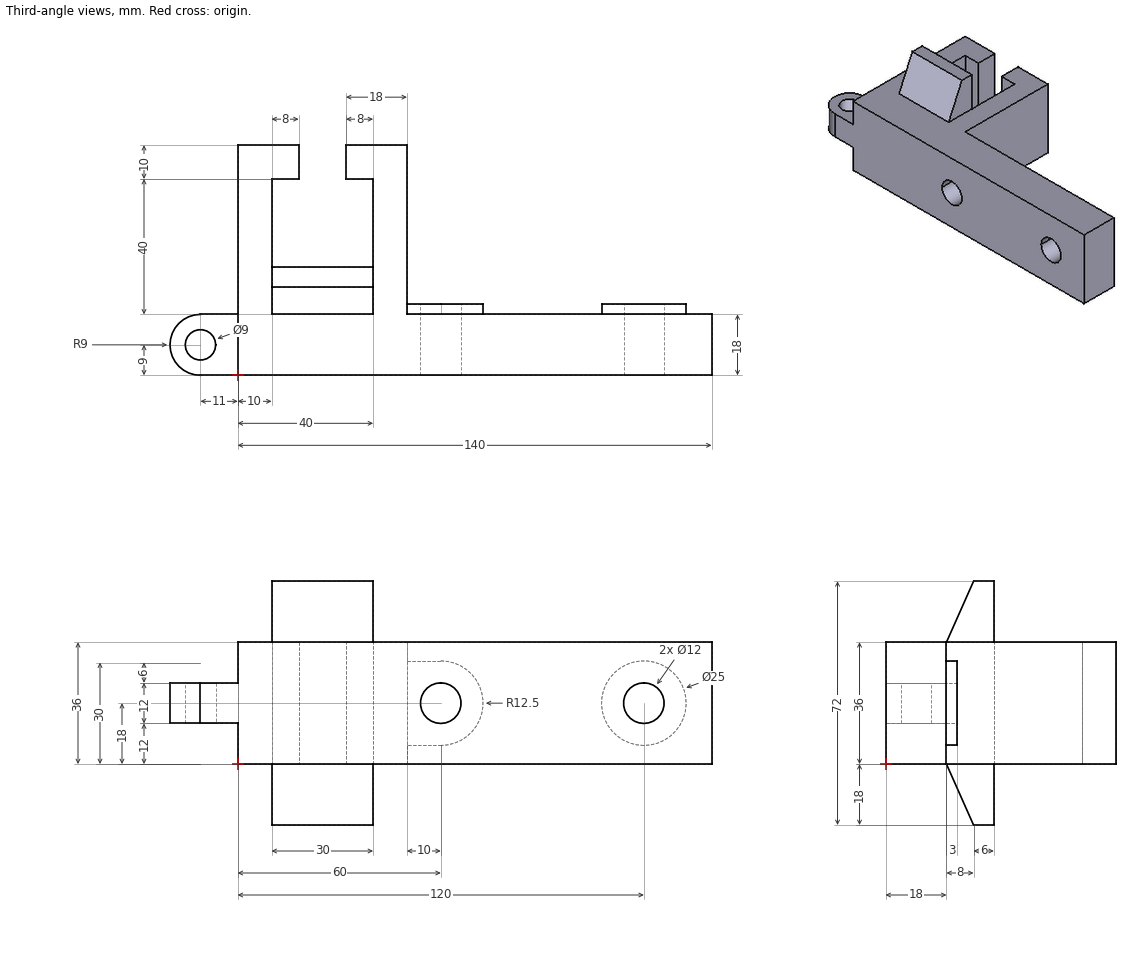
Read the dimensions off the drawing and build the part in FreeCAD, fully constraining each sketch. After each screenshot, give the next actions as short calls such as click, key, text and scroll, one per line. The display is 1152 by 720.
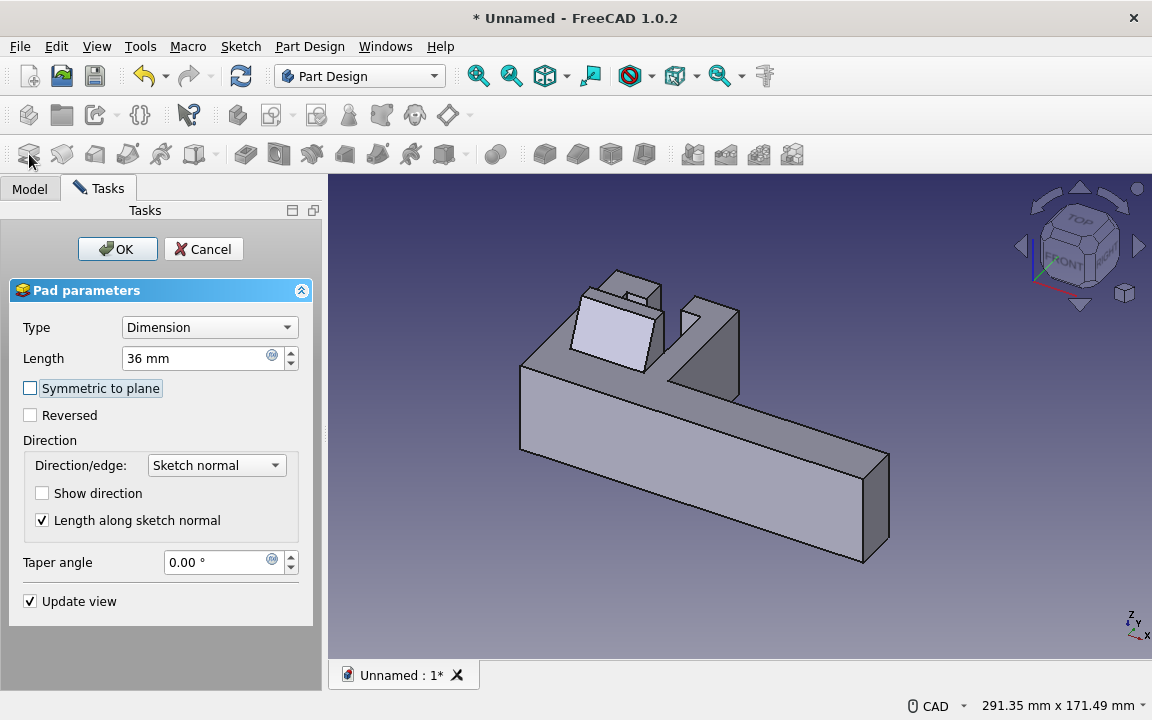
click(118, 249)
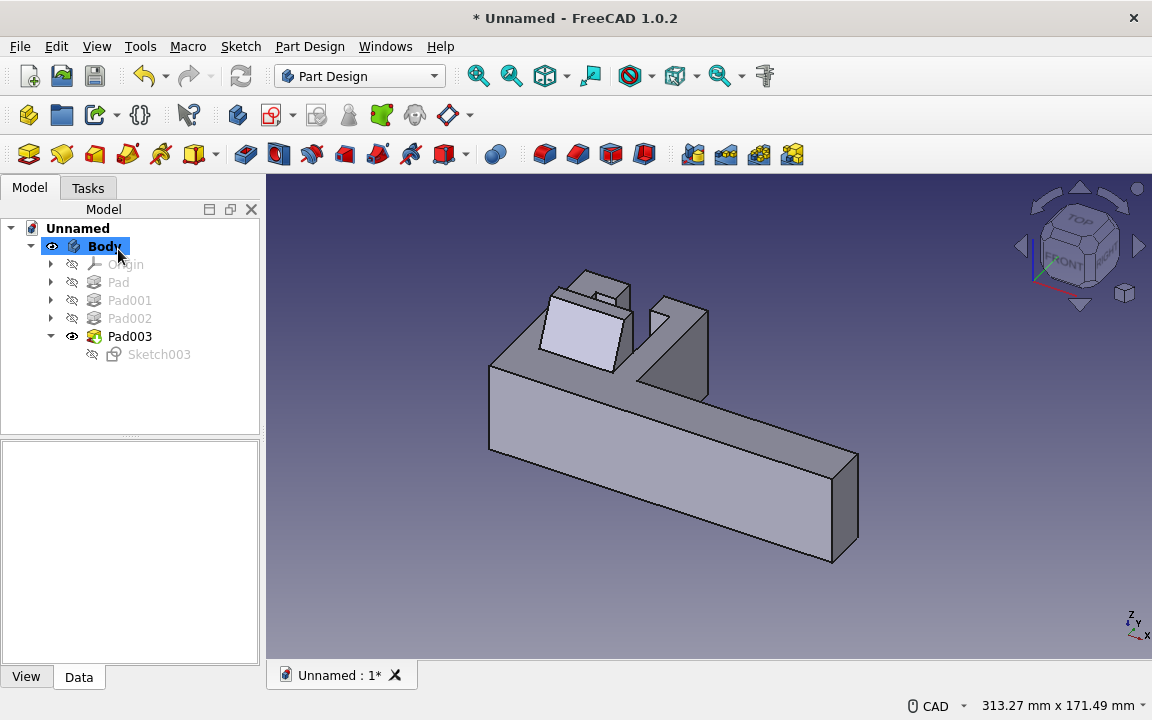
key(5)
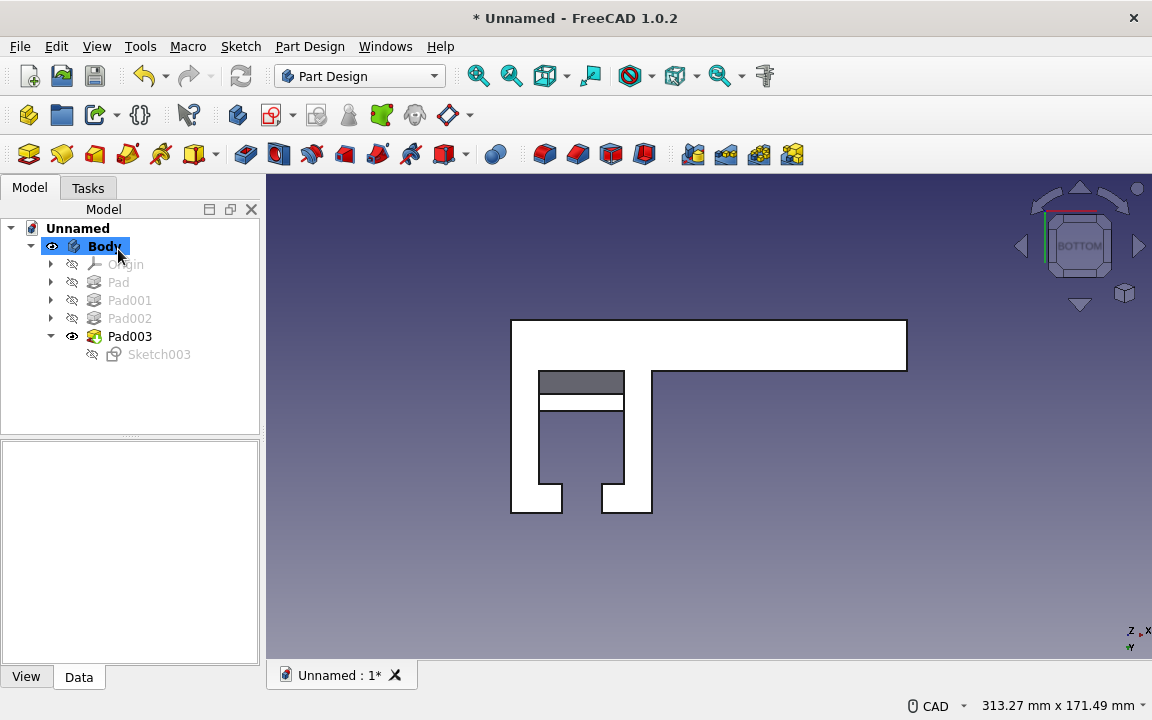
key(v)
key(f)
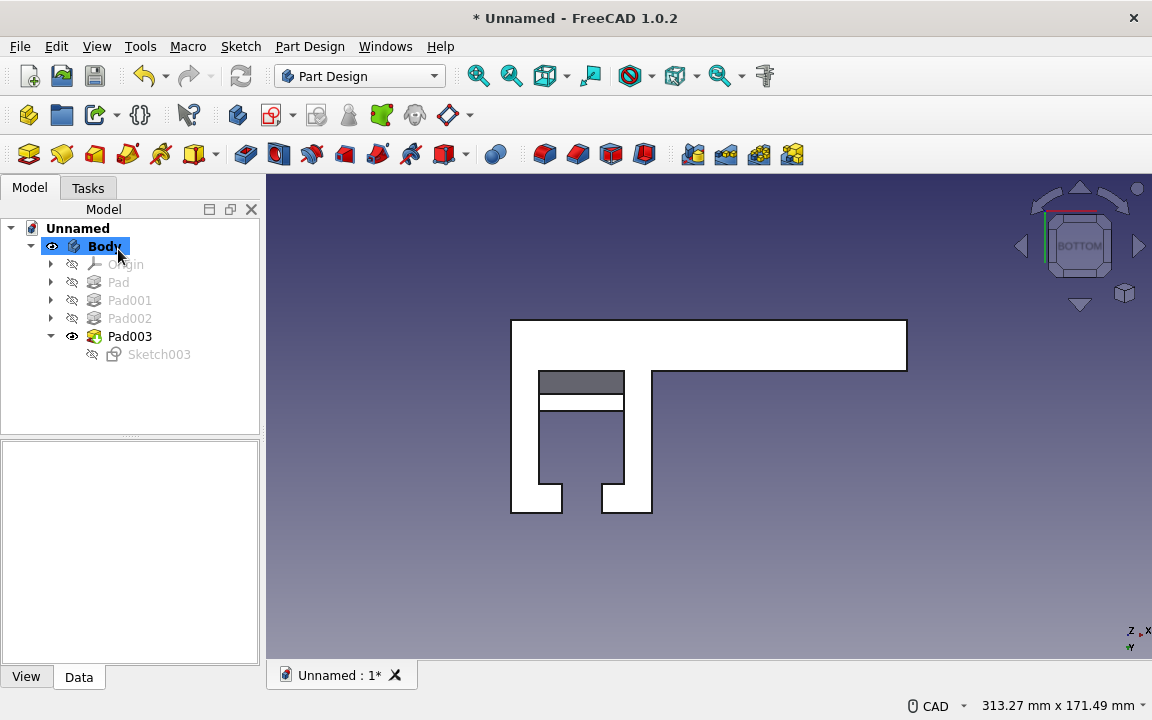
click(879, 333)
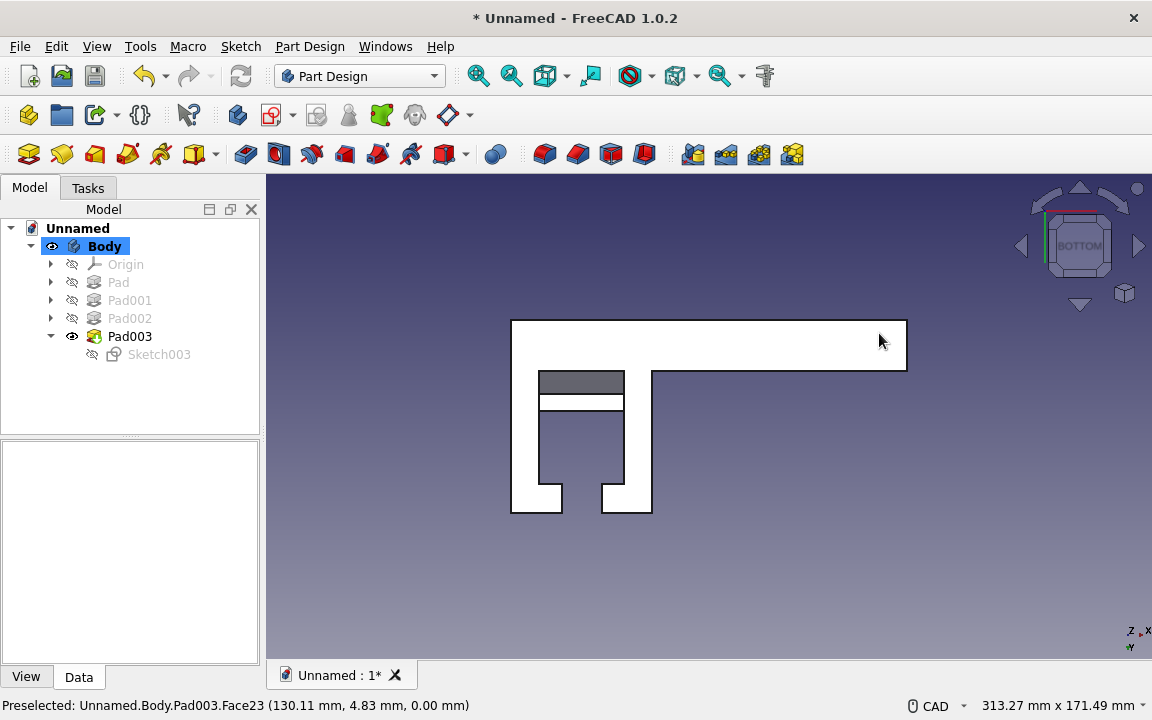
click(270, 116)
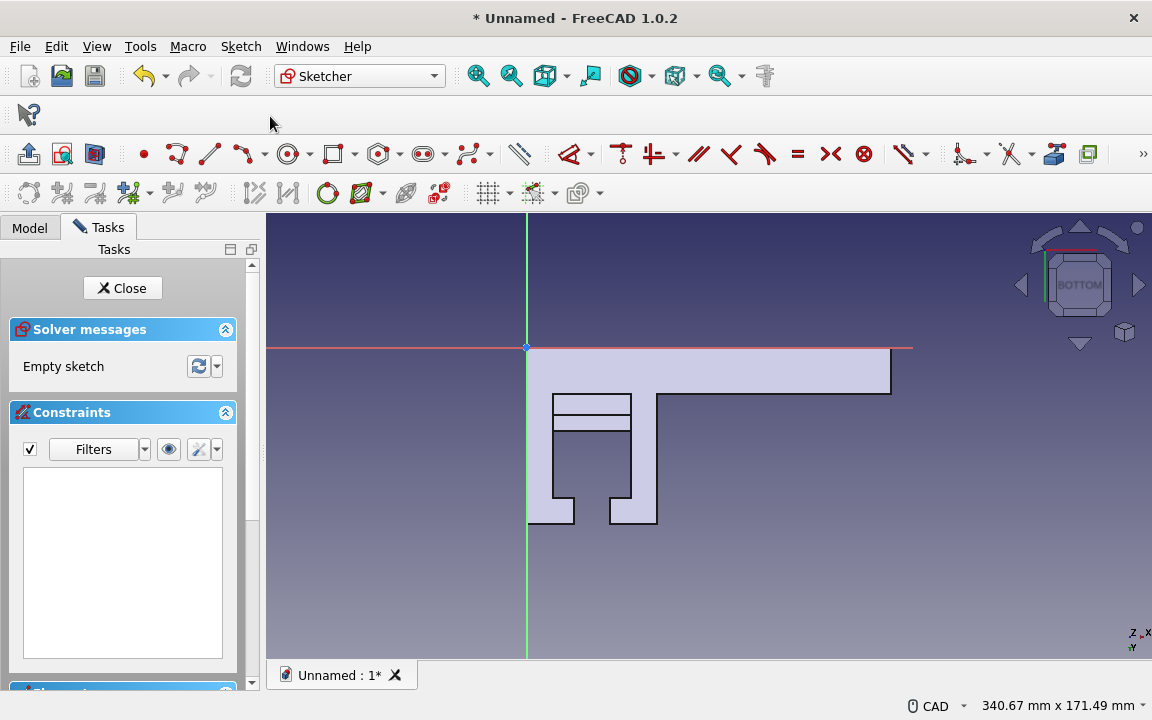
key(q)
key(s)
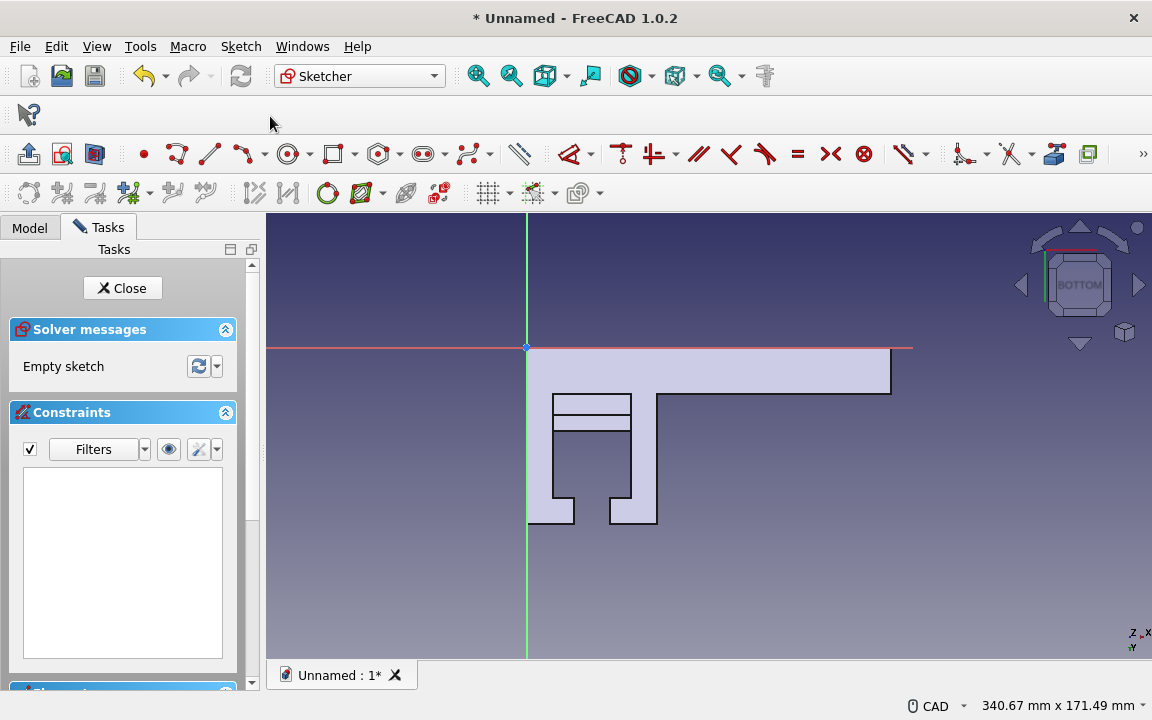
scroll(473, 358, up, 9)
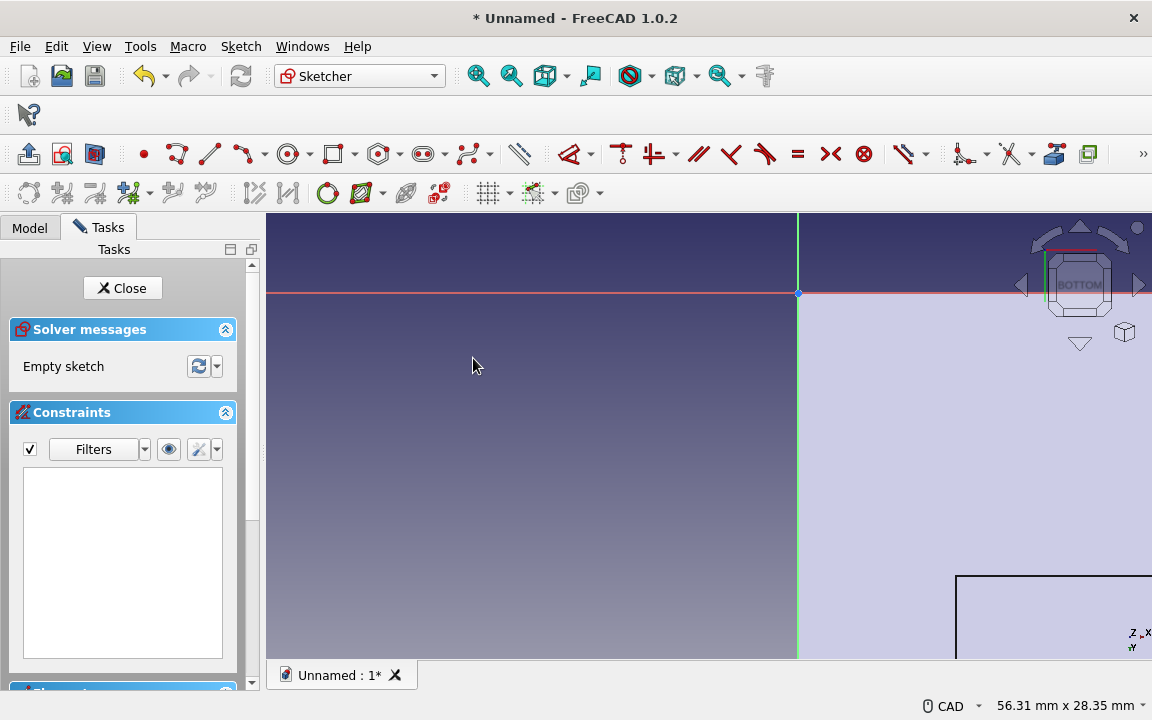
click(177, 154)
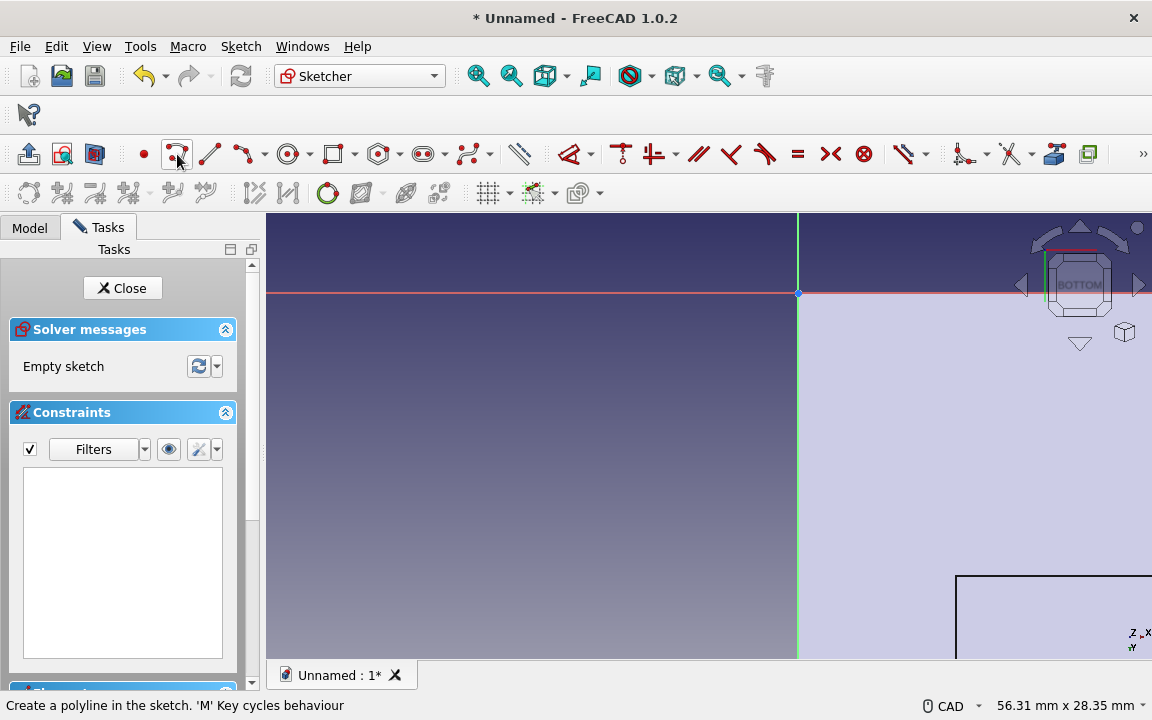
click(625, 576)
click(798, 576)
click(798, 293)
click(625, 302)
right_click(625, 302)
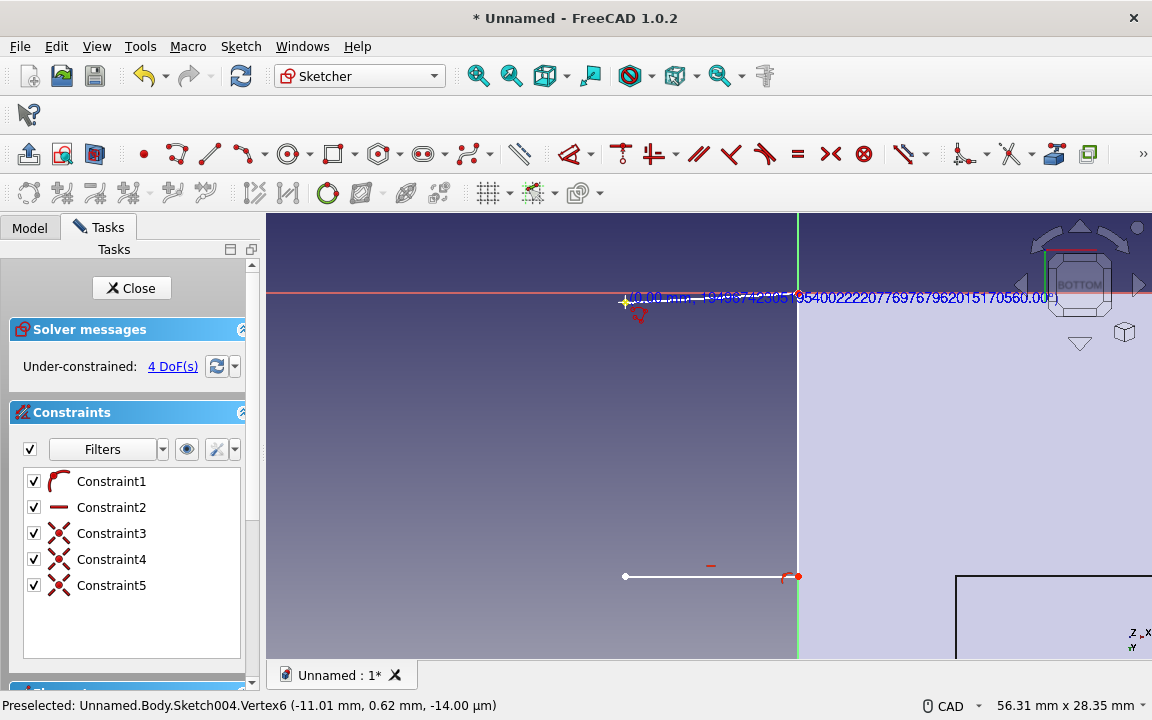
key(g)
key(3)
key(a)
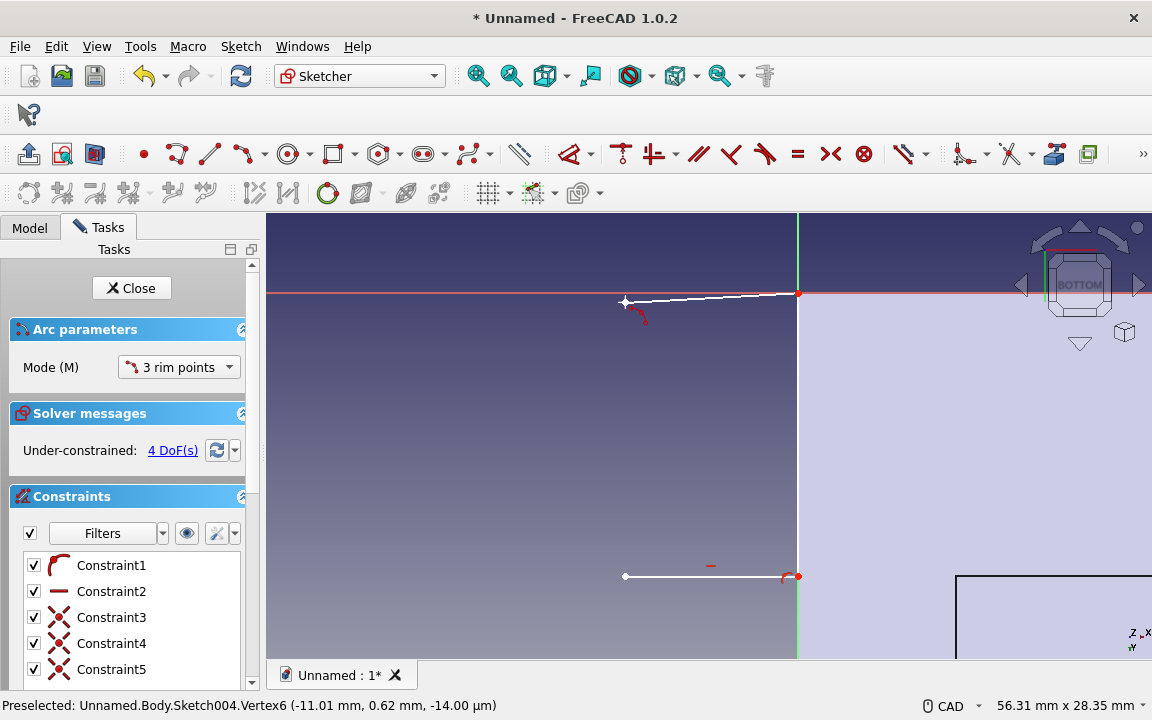
click(625, 303)
click(625, 577)
click(483, 435)
key(Escape)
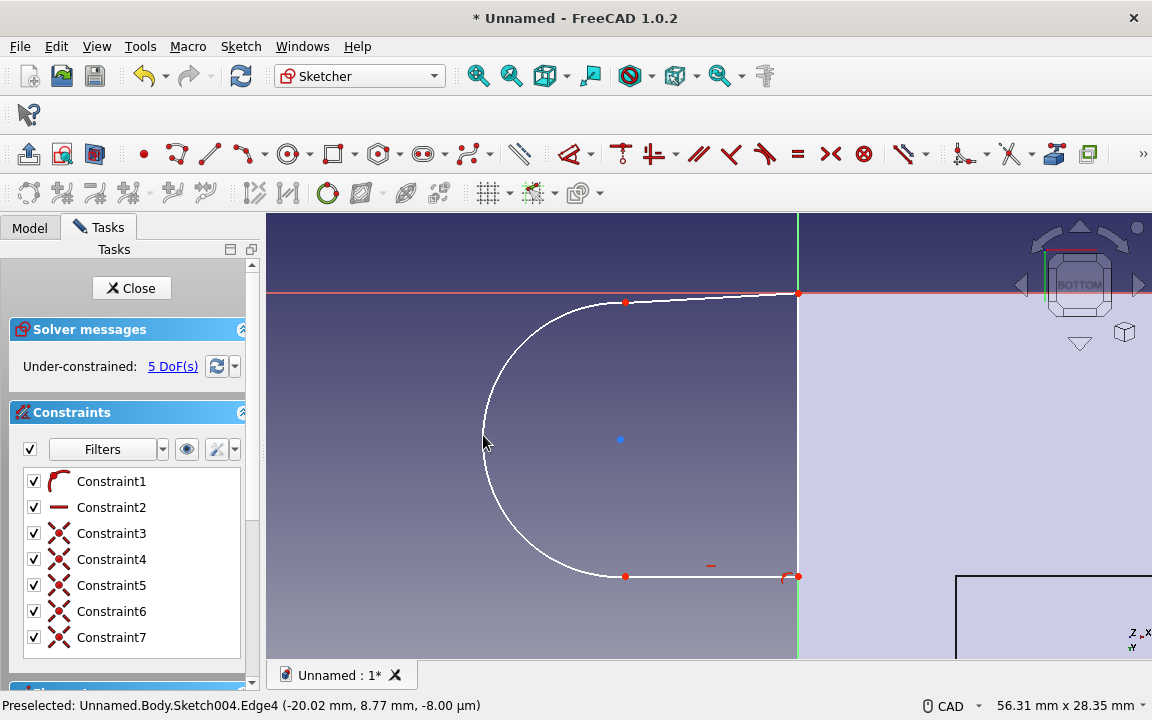
click(677, 577)